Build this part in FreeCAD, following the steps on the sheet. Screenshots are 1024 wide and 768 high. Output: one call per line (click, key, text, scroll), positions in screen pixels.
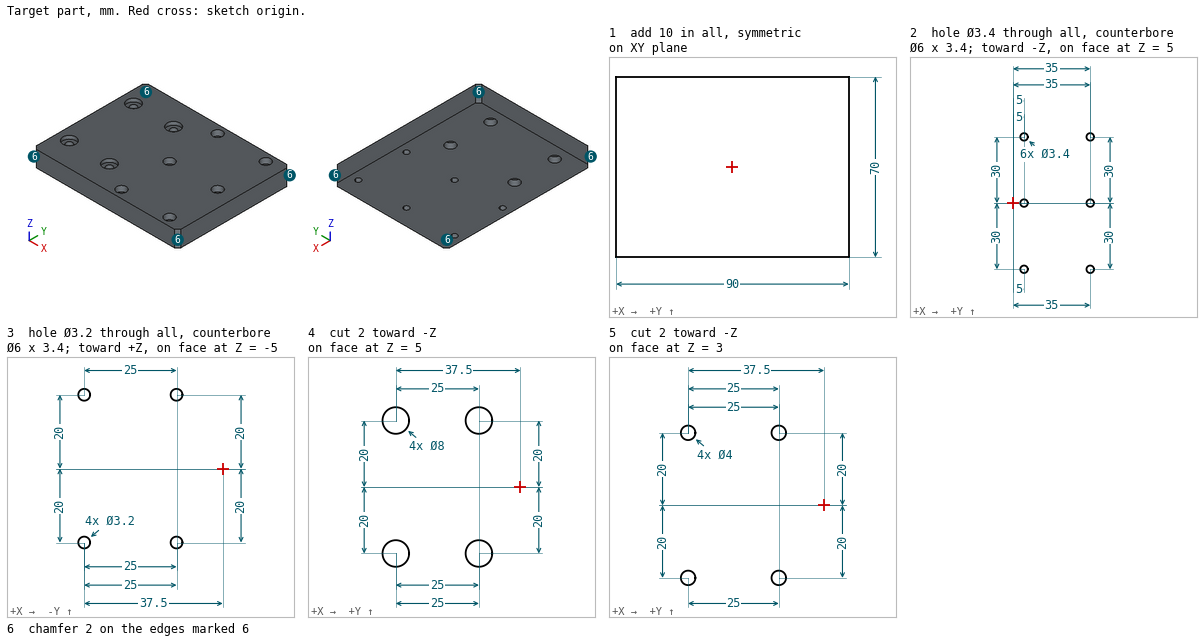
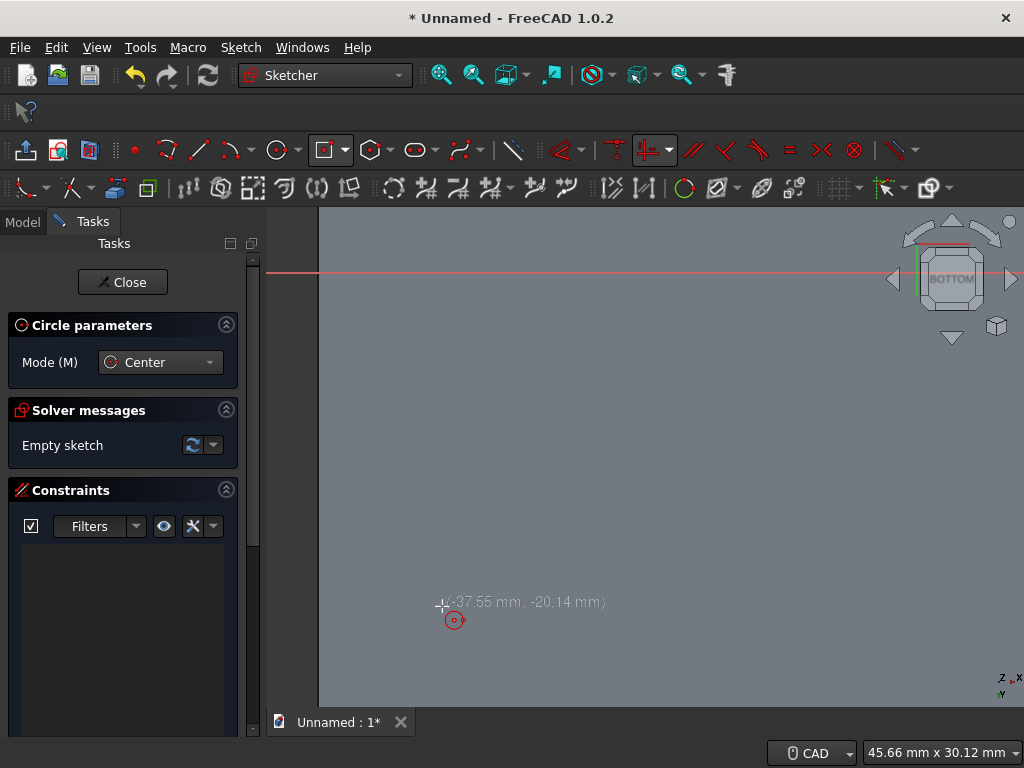
click(443, 605)
click(461, 586)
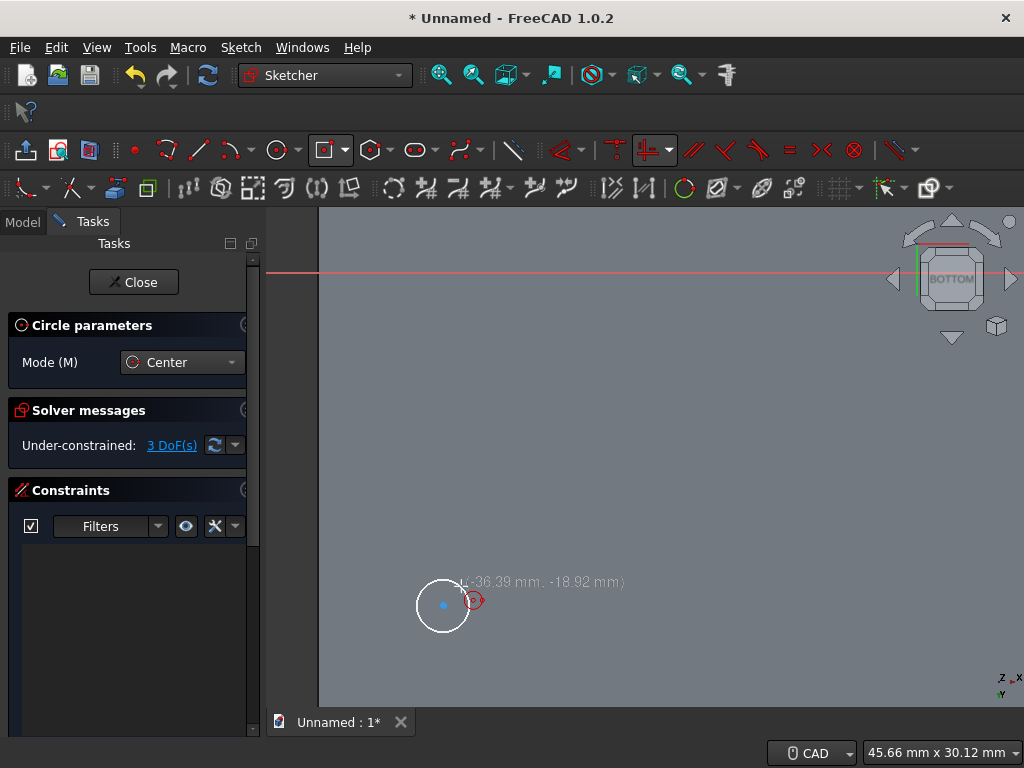
click(858, 605)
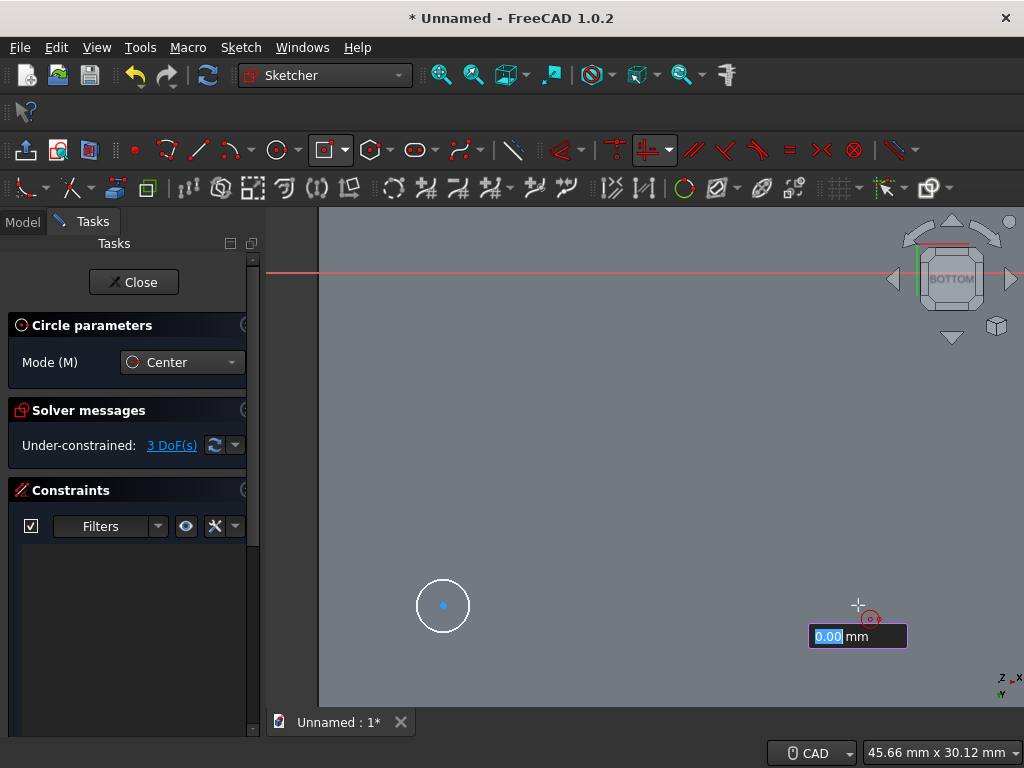
scroll(443, 607, down, 4)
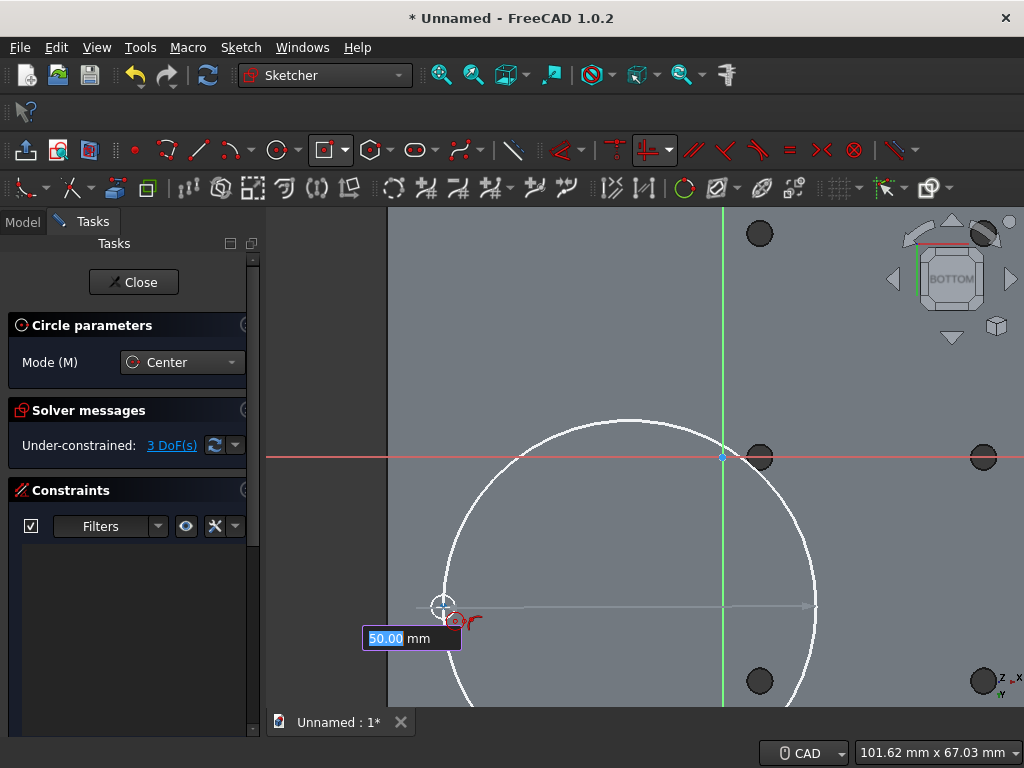
scroll(638, 598, up, 2)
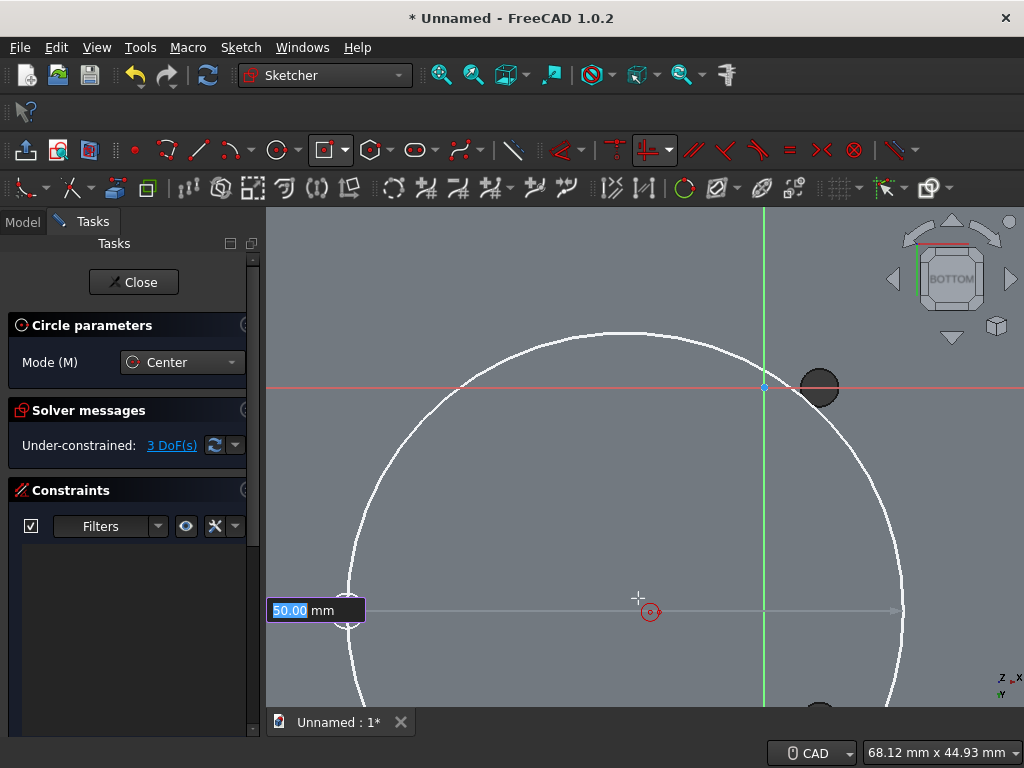
click(637, 598)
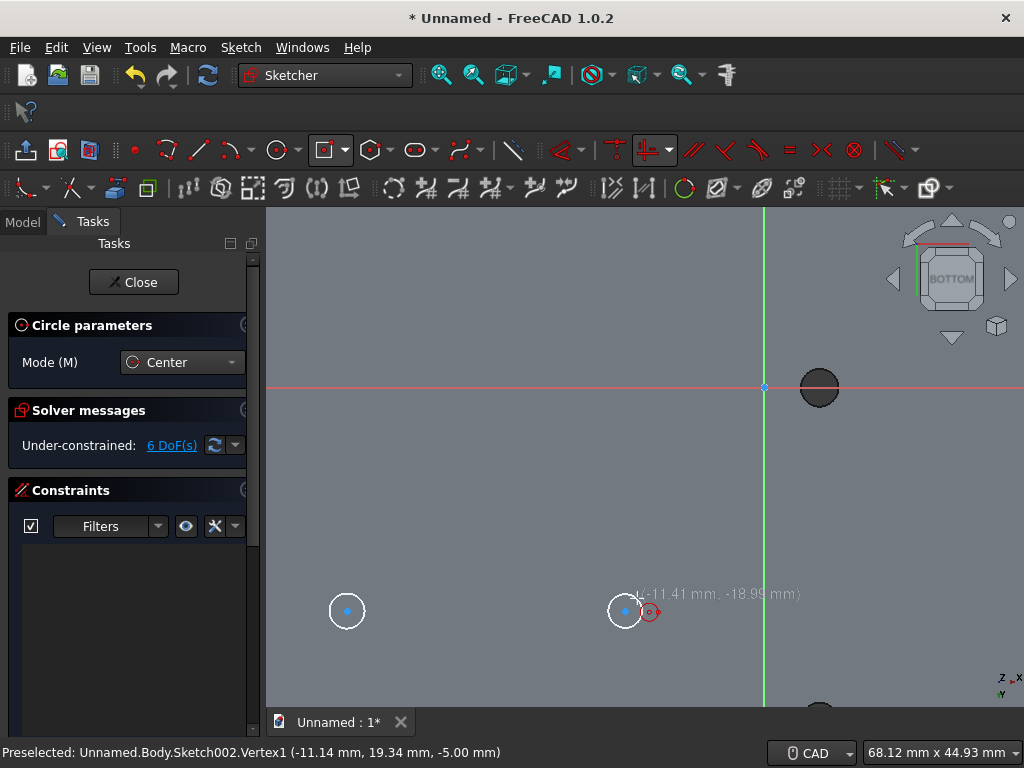
scroll(638, 598, down, 2)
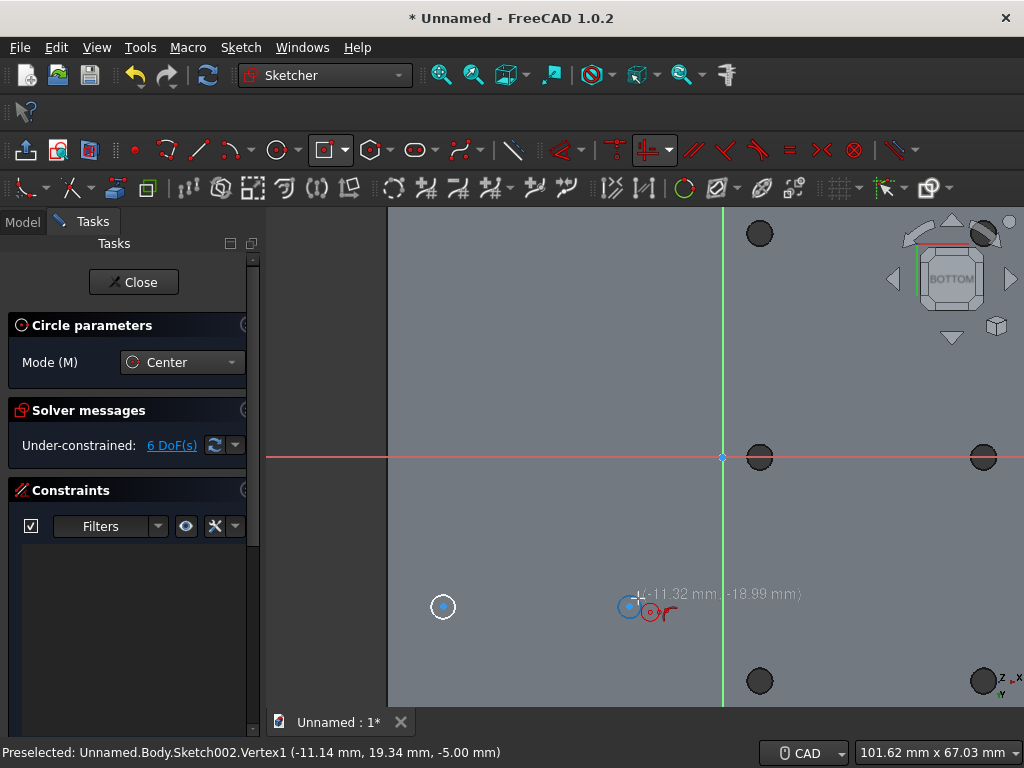
scroll(629, 308, up, 4)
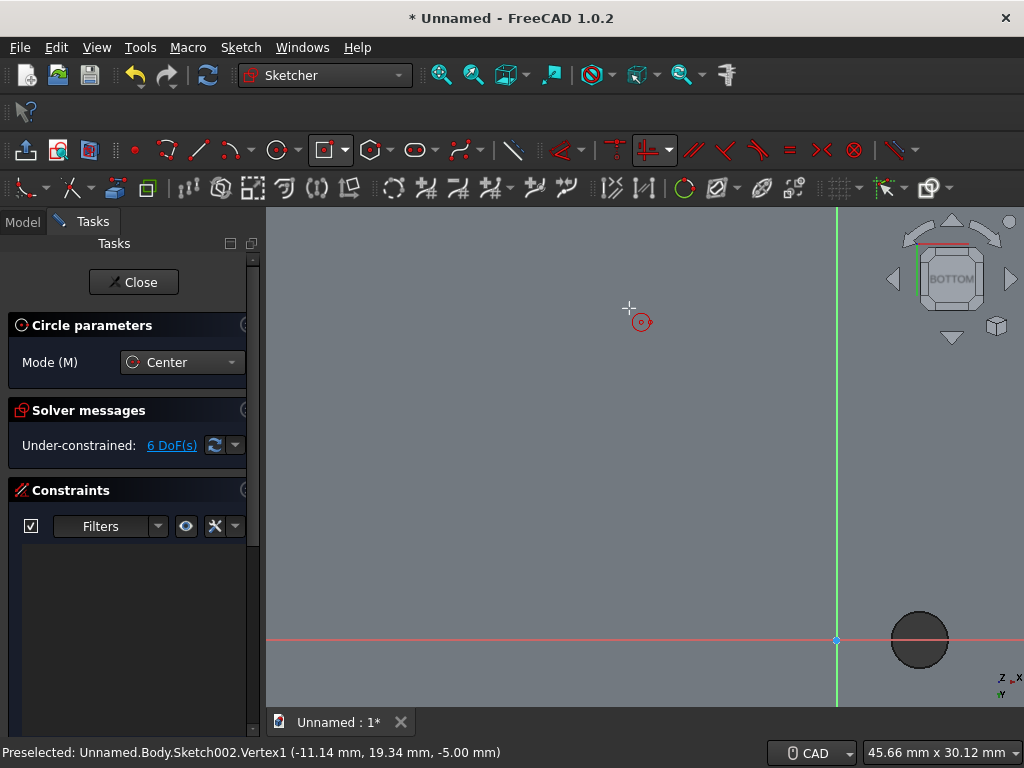
click(629, 308)
click(648, 289)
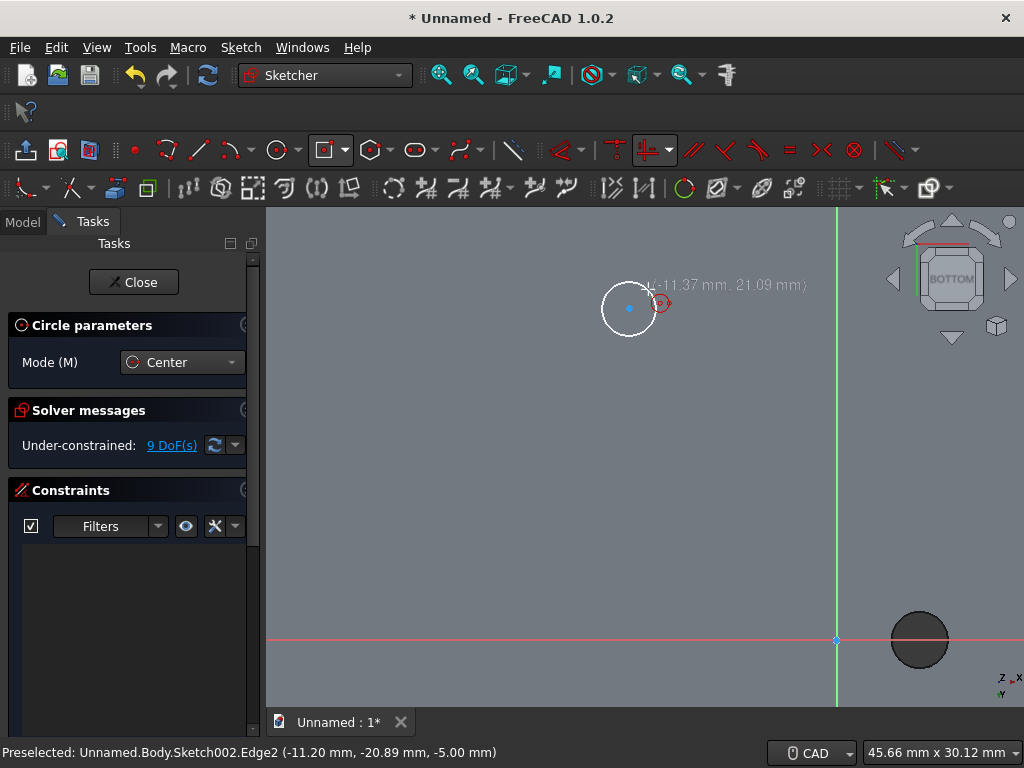
scroll(629, 308, down, 4)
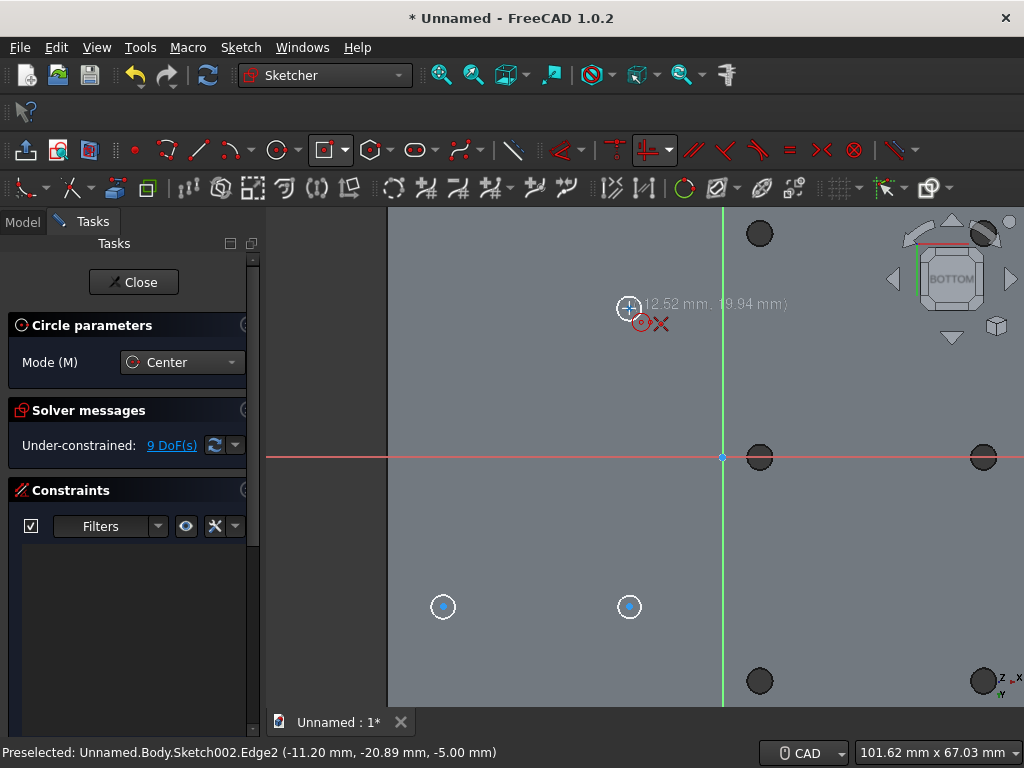
scroll(443, 308, up, 4)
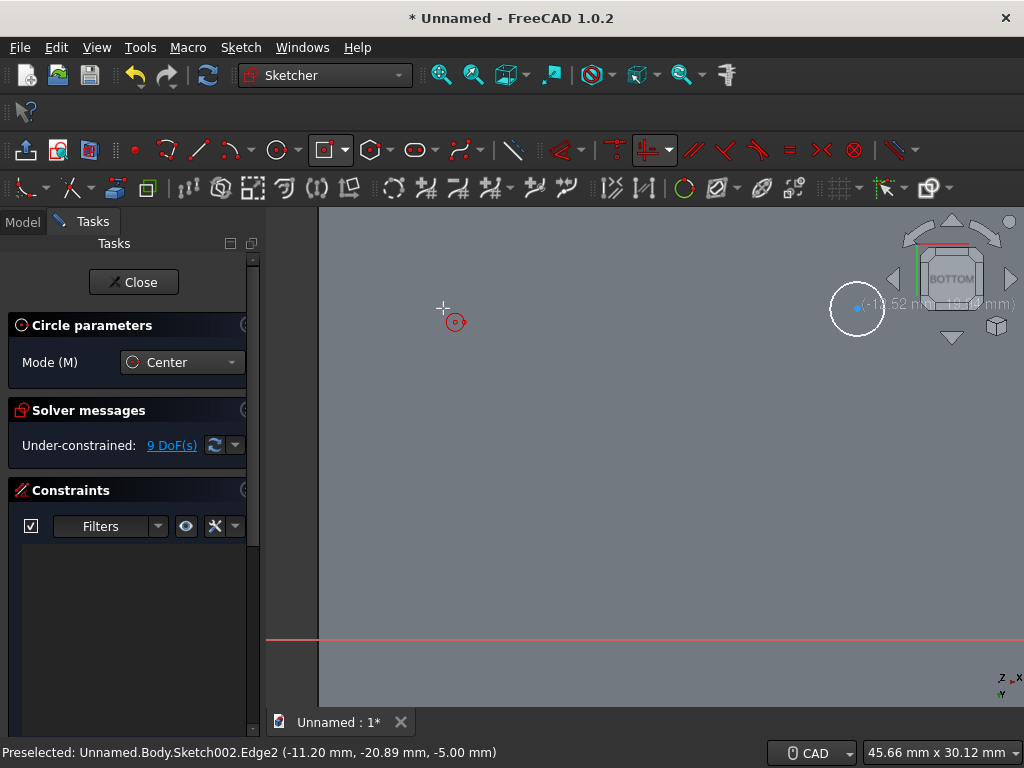
click(443, 308)
click(461, 289)
key(Escape)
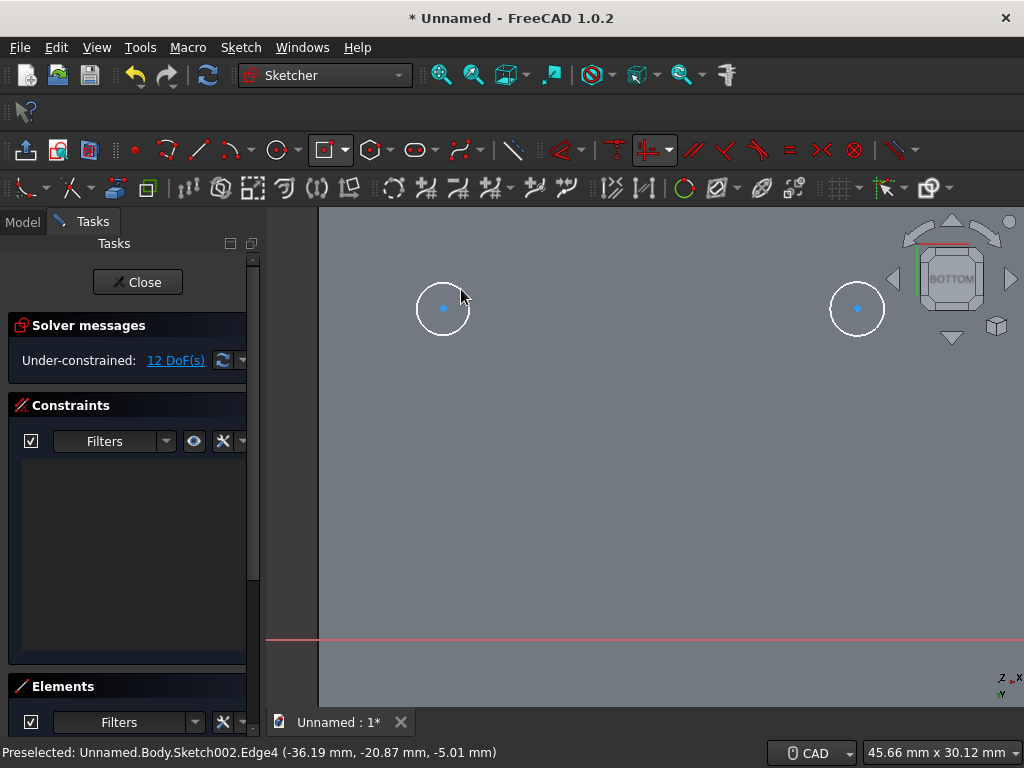
scroll(443, 308, down, 4)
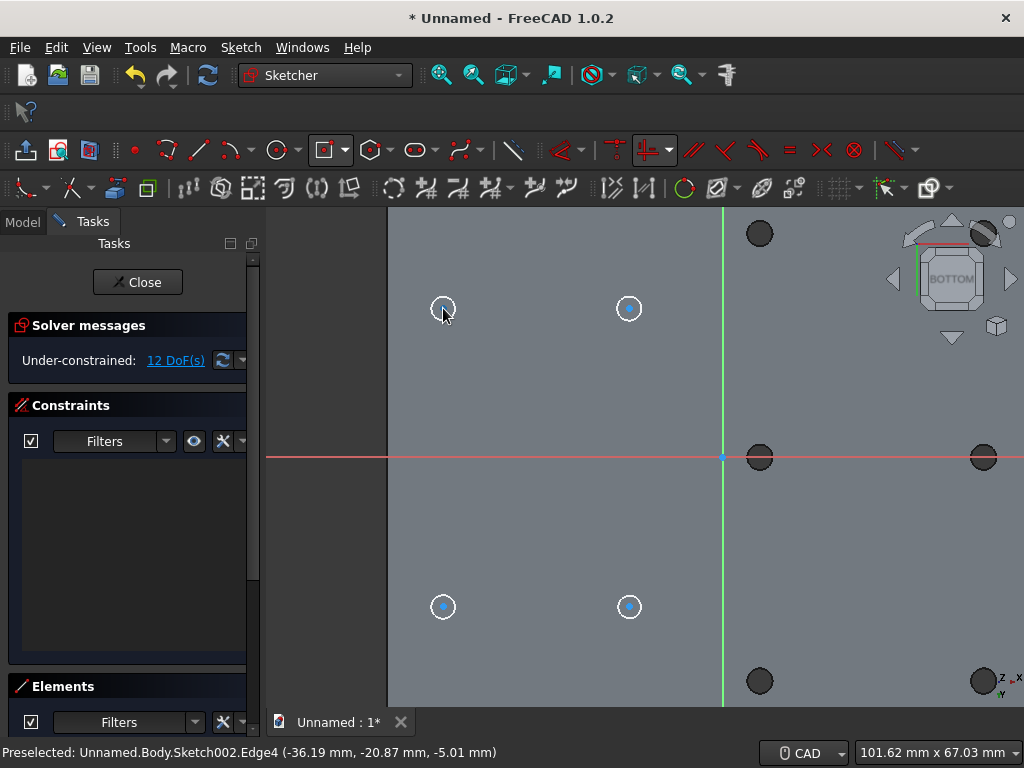
click(451, 599)